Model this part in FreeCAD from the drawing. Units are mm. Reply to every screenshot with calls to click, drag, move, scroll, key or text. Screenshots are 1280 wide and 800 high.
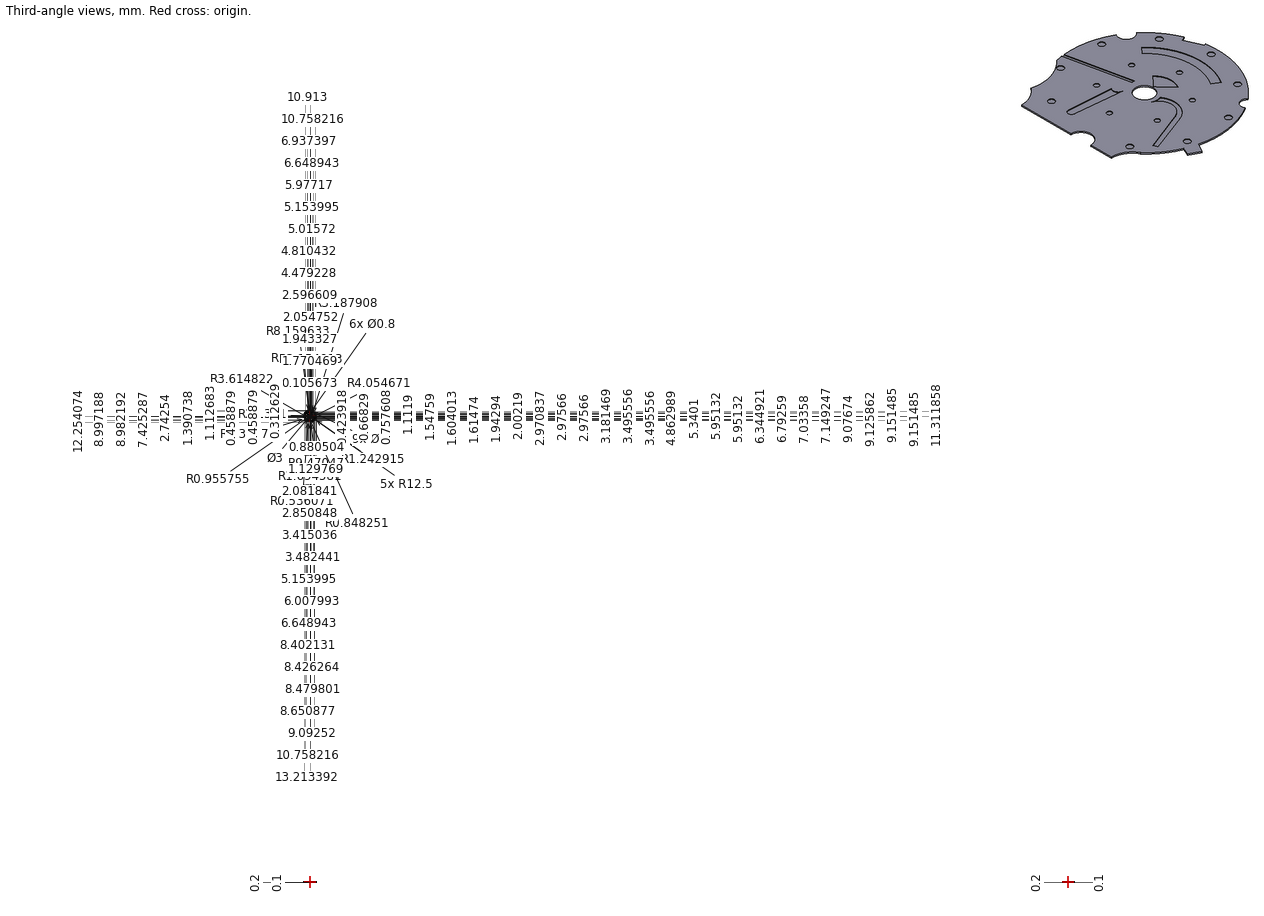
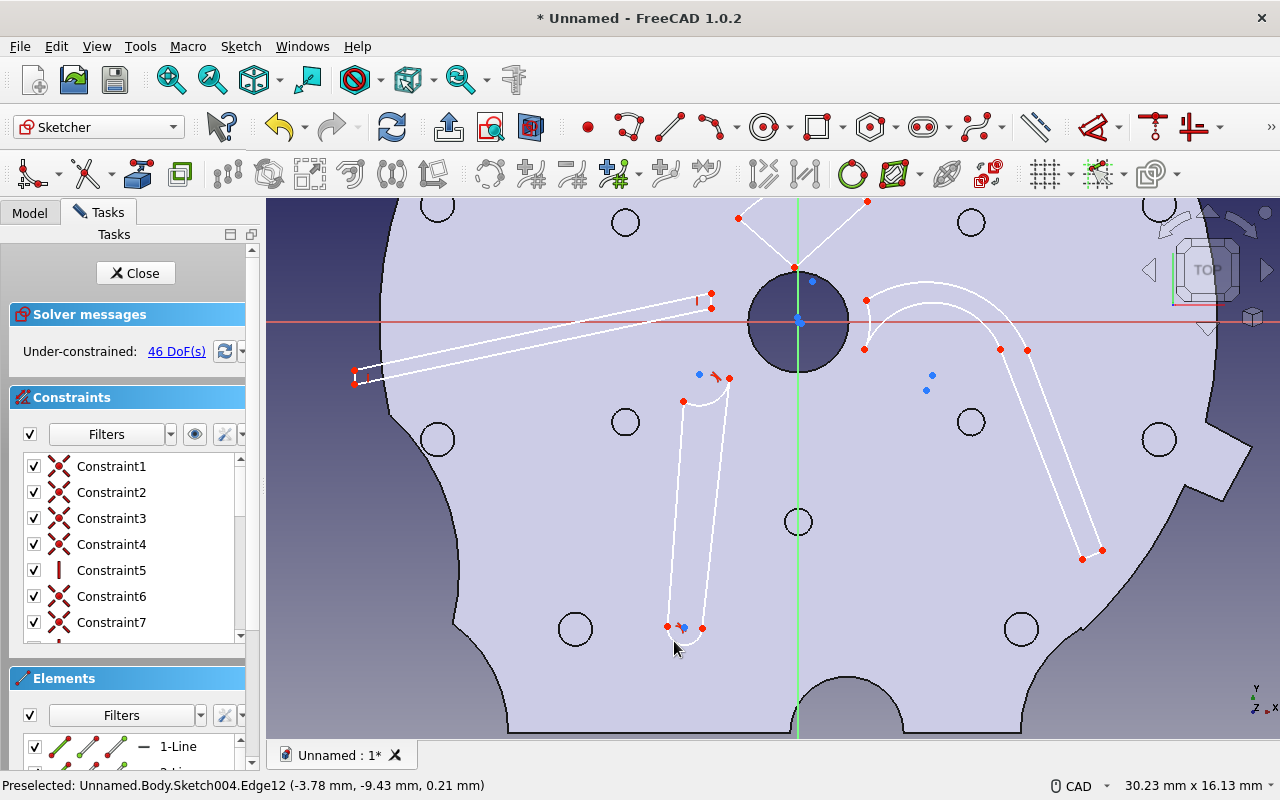
click(1025, 412)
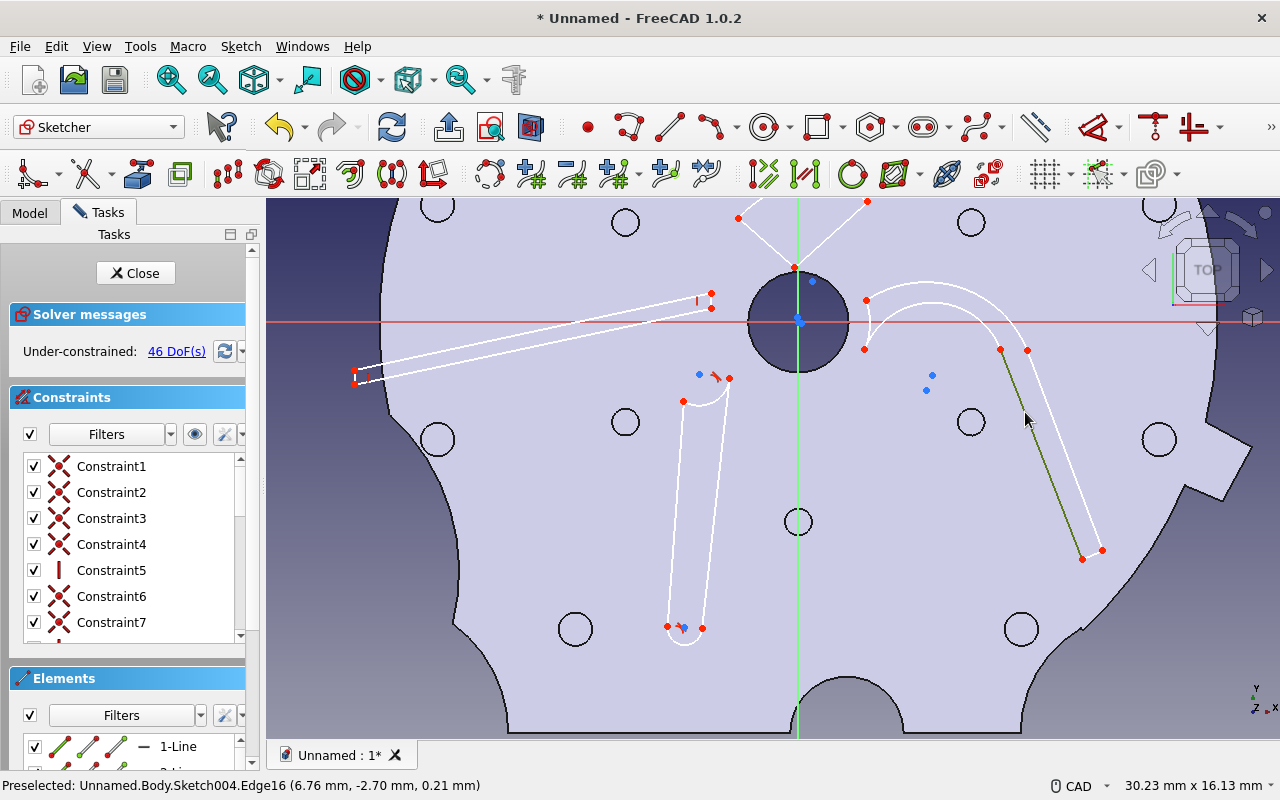
click(966, 311)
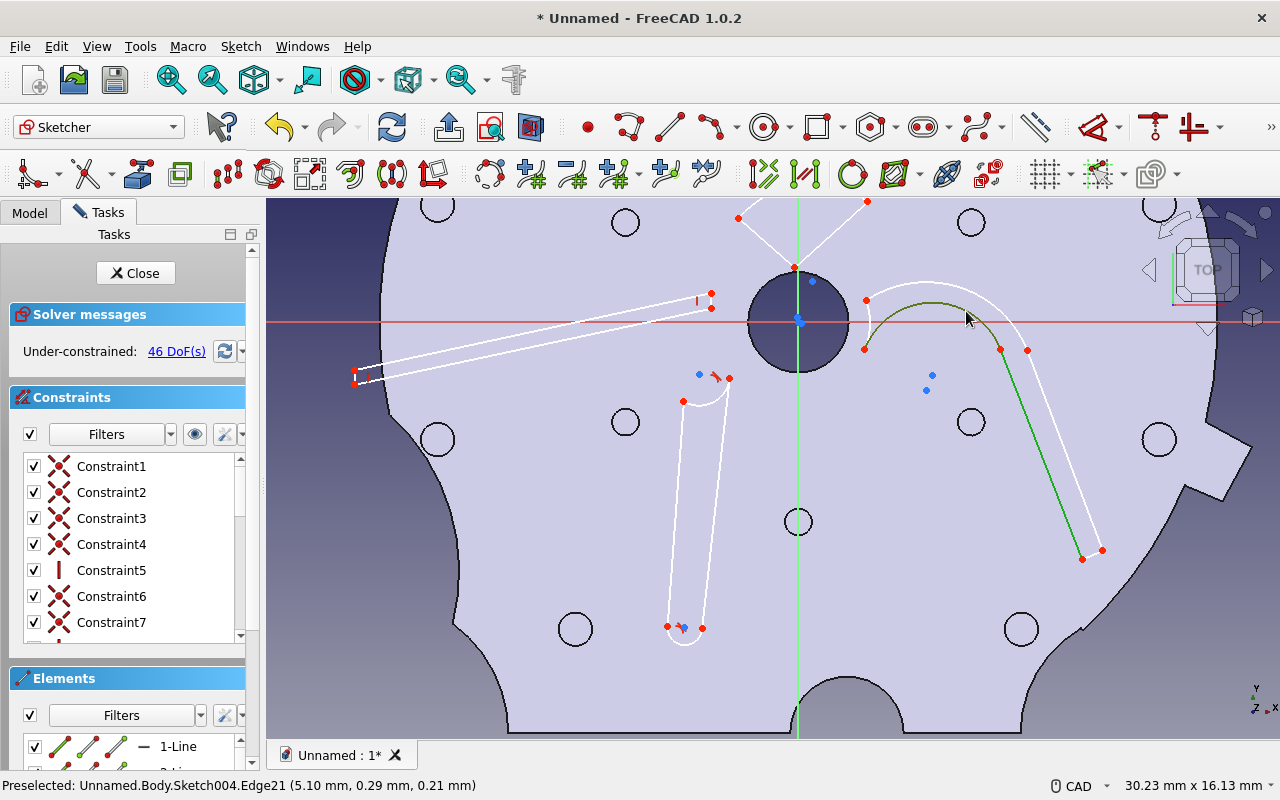
key(t)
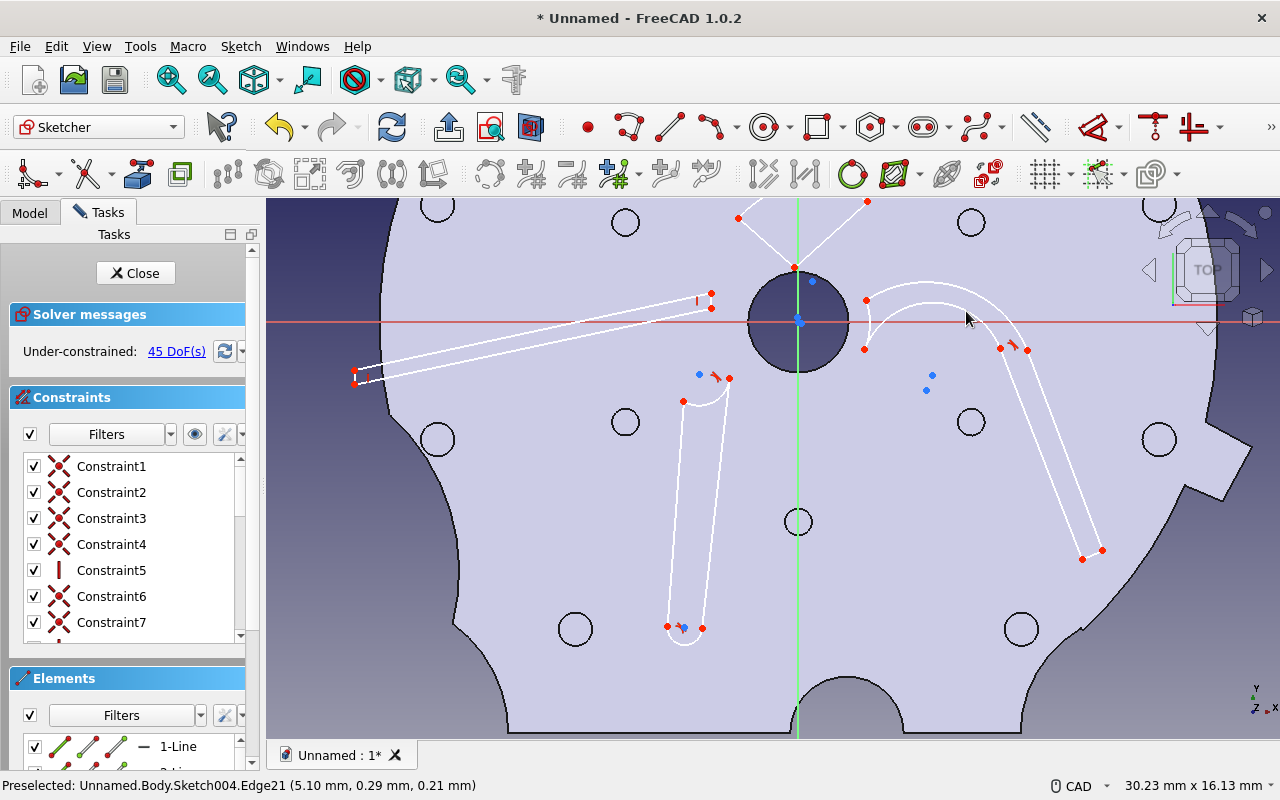
click(1080, 491)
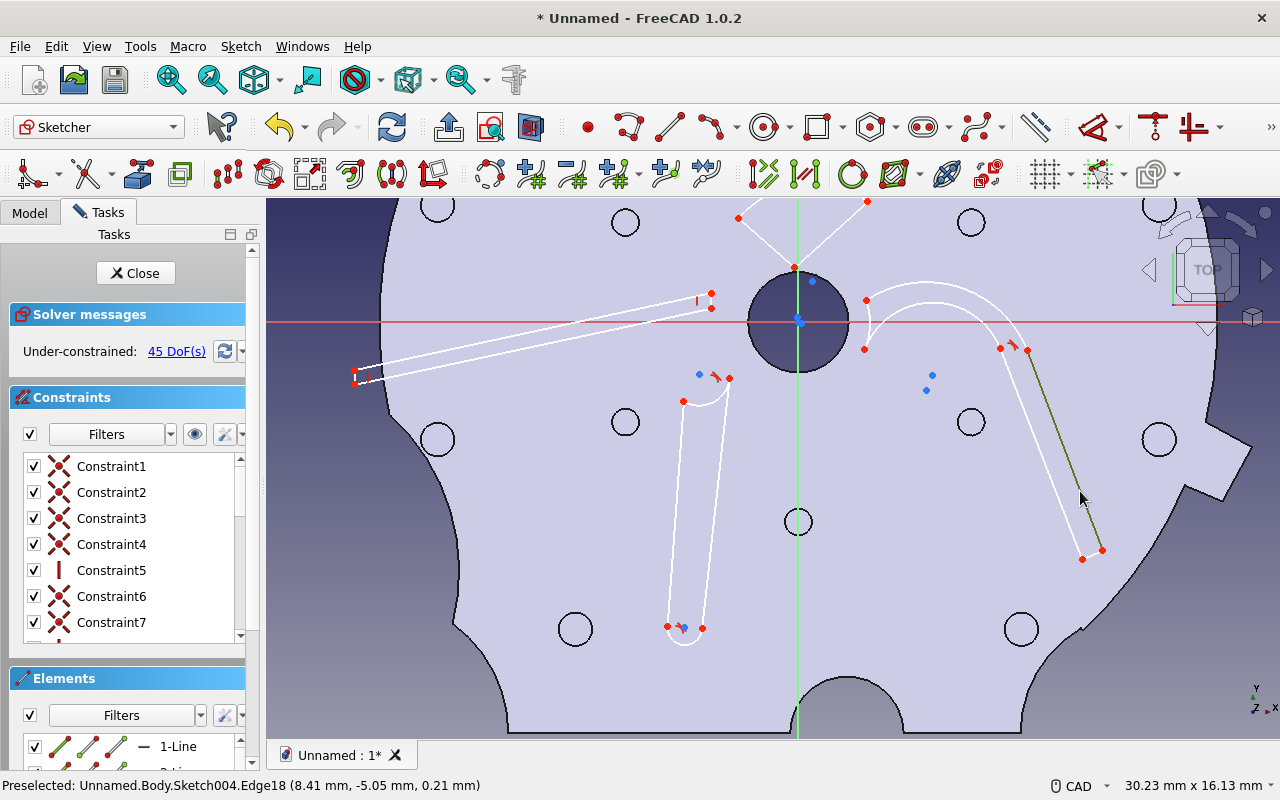
click(993, 305)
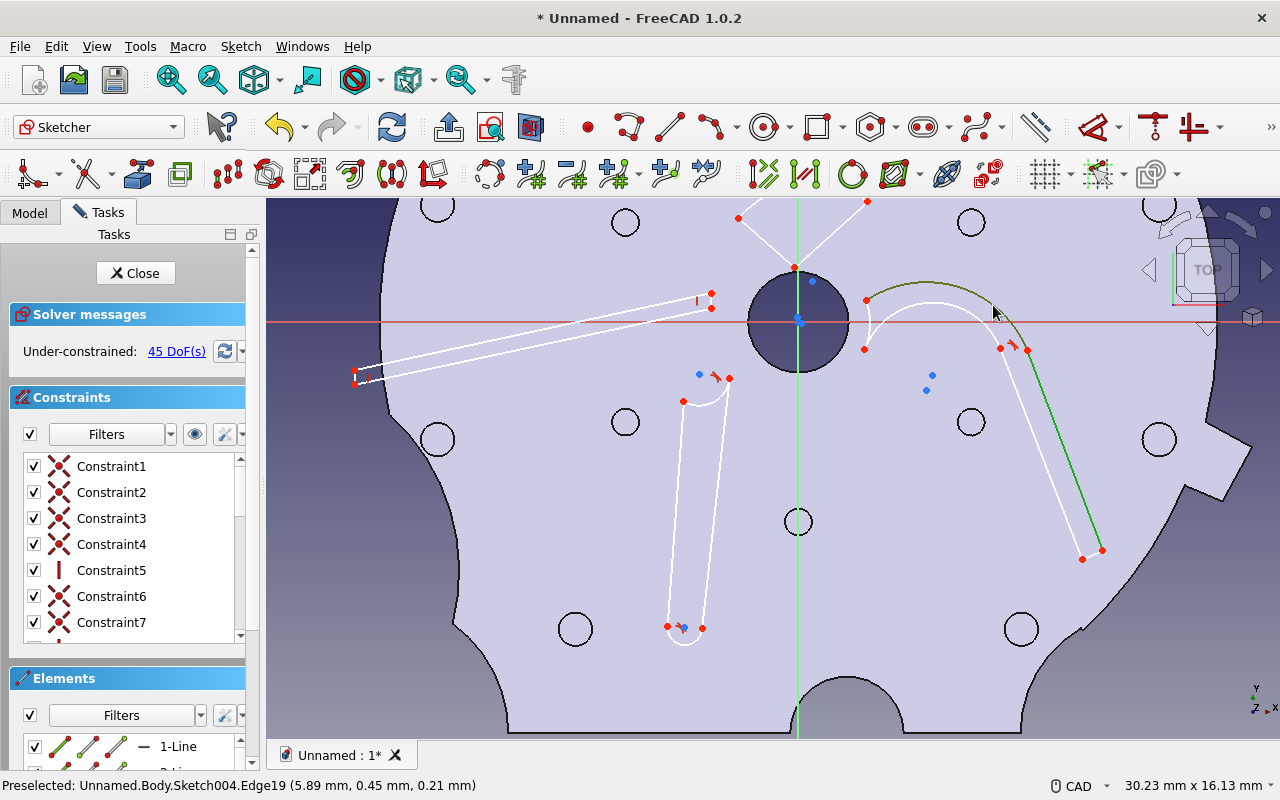
key(t)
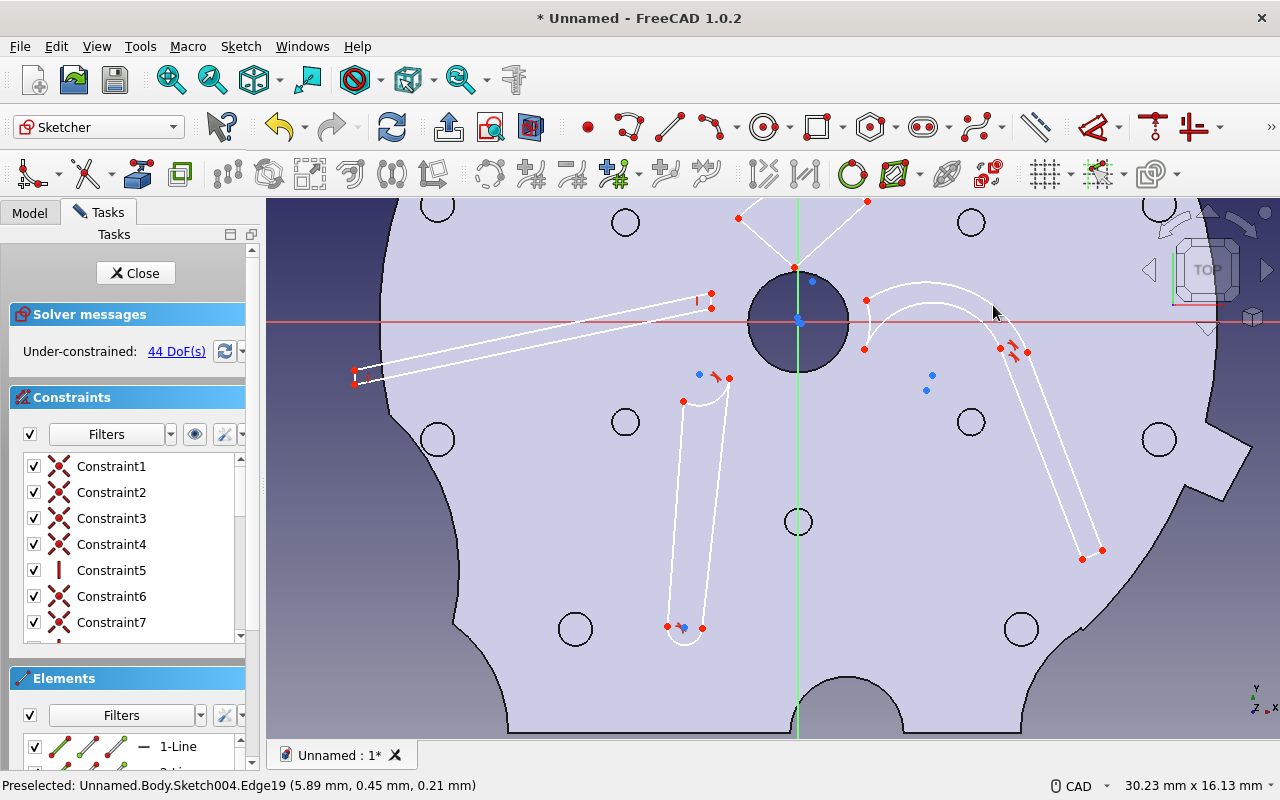
scroll(869, 310, up, 2)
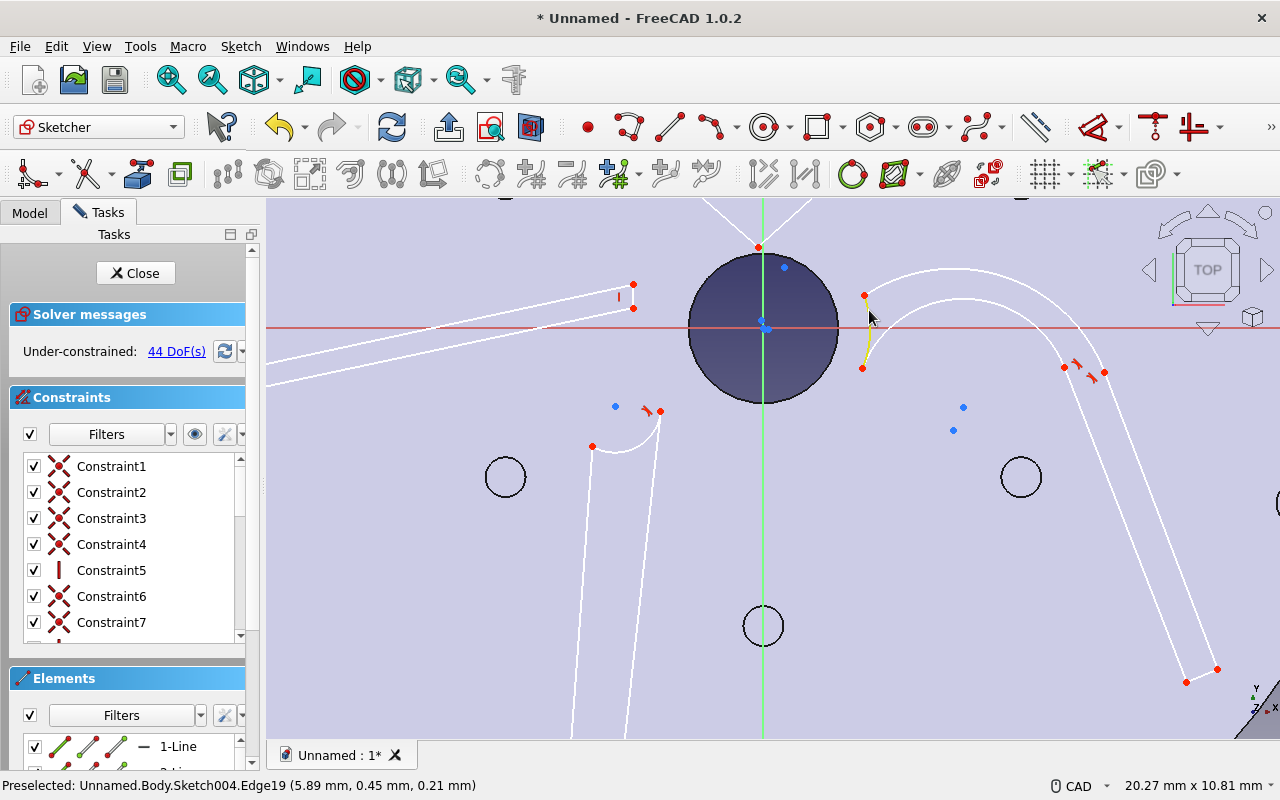
click(868, 310)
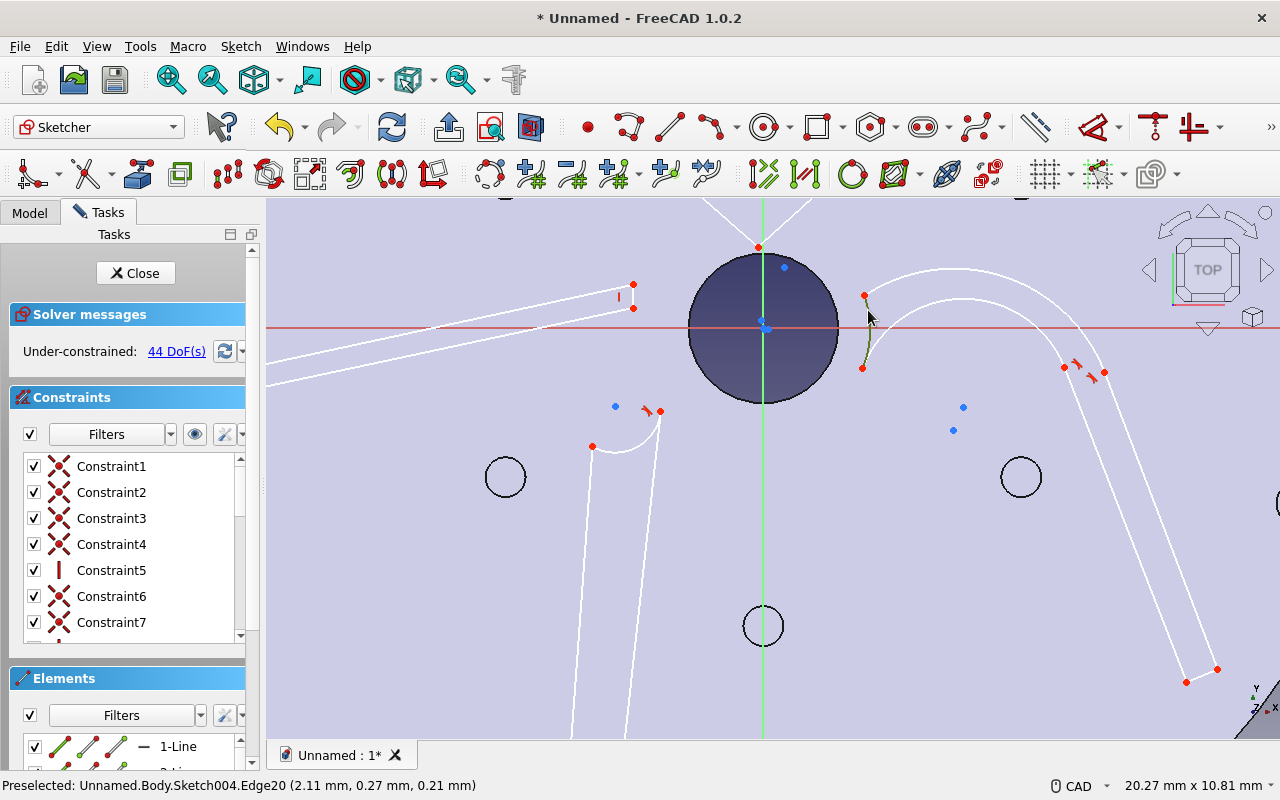
click(1014, 311)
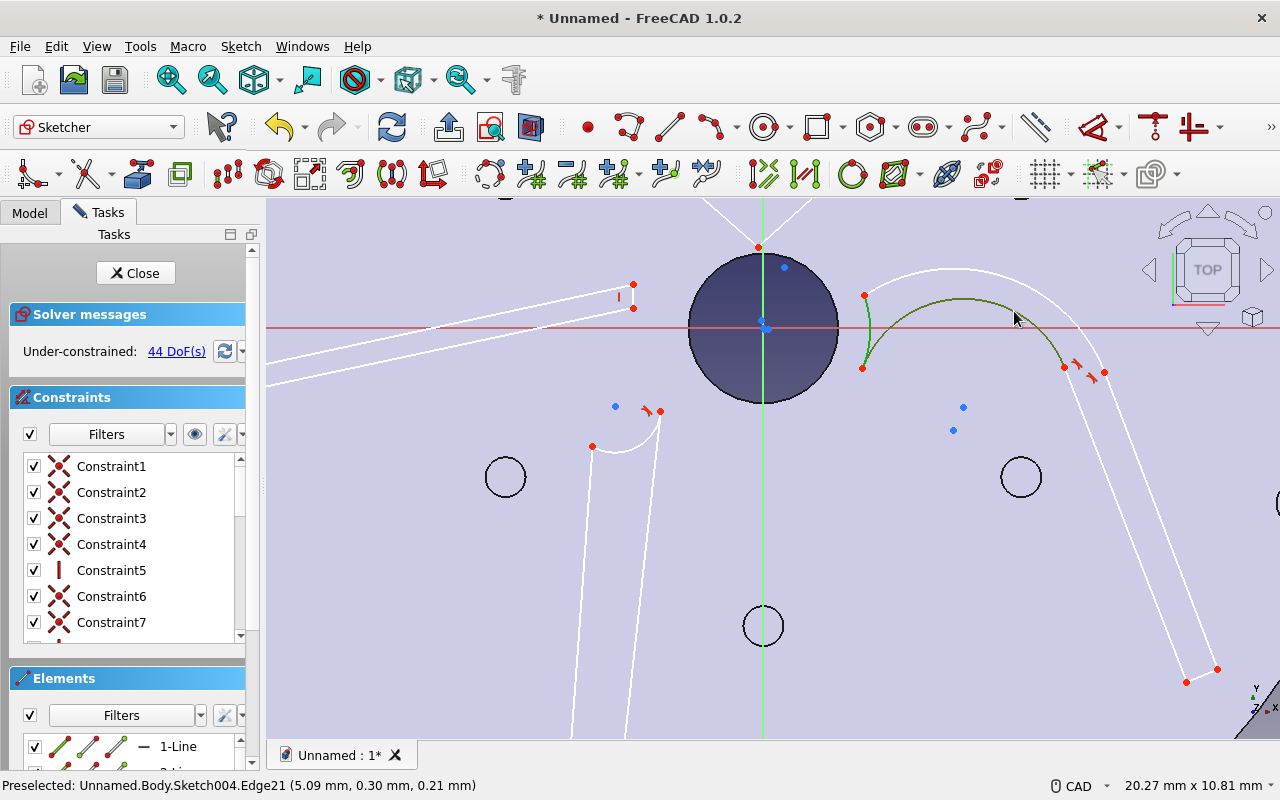
key(t)